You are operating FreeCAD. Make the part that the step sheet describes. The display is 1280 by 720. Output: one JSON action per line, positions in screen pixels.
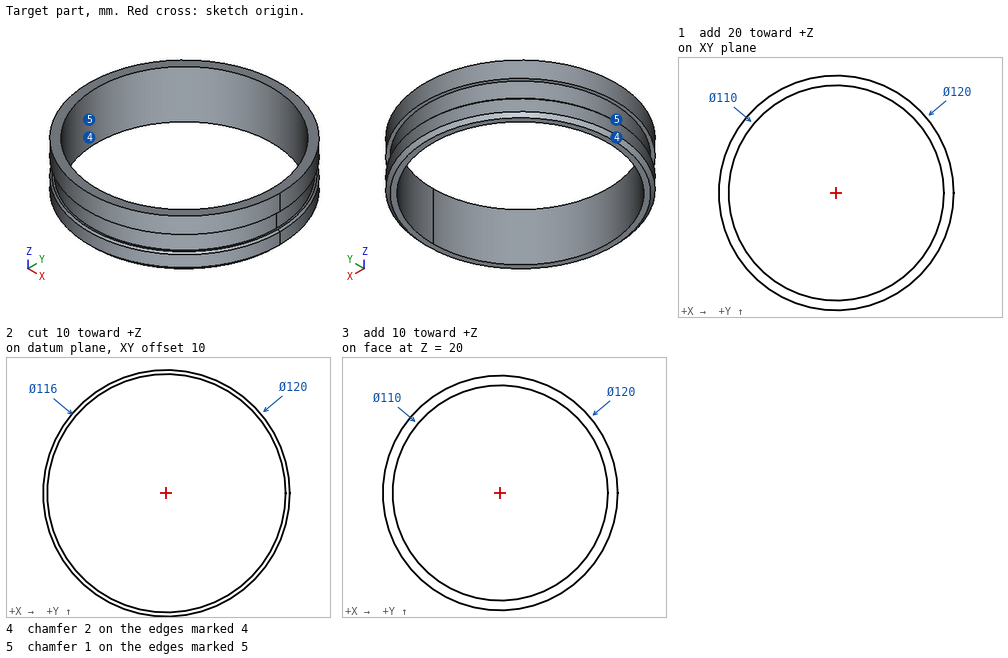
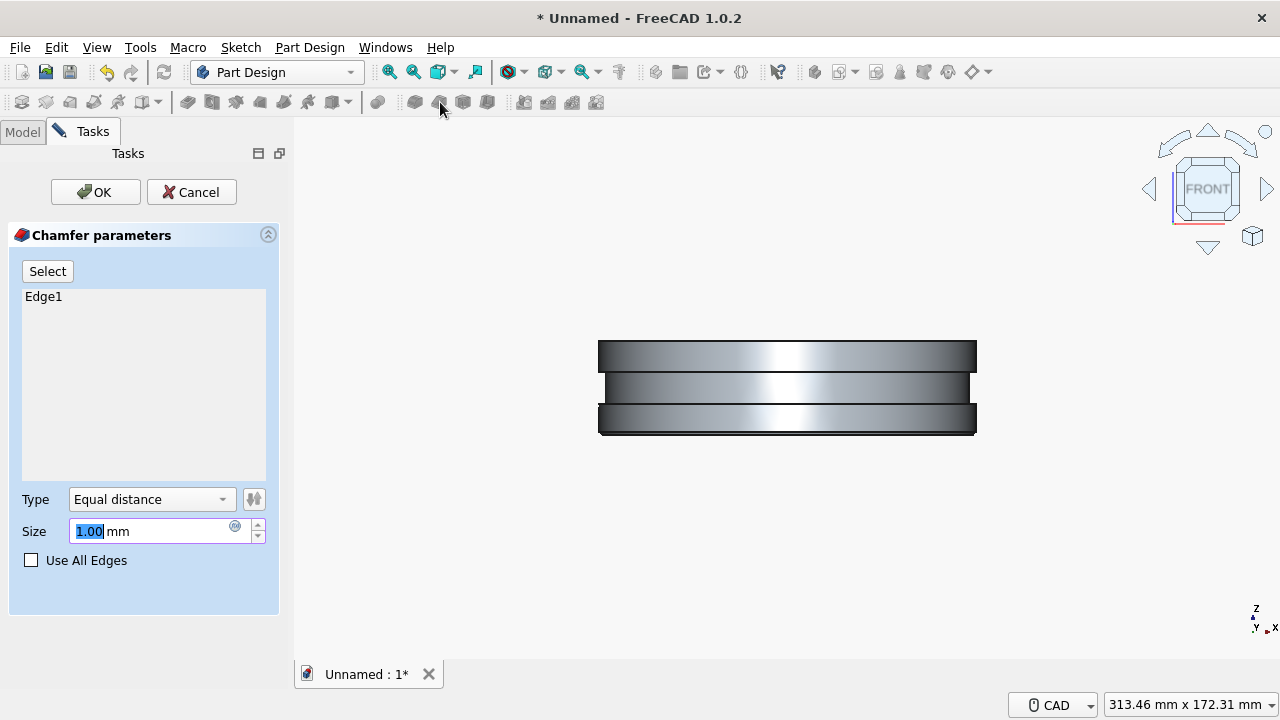
{"action": "type", "text": "2"}
{"action": "key", "text": "Tab"}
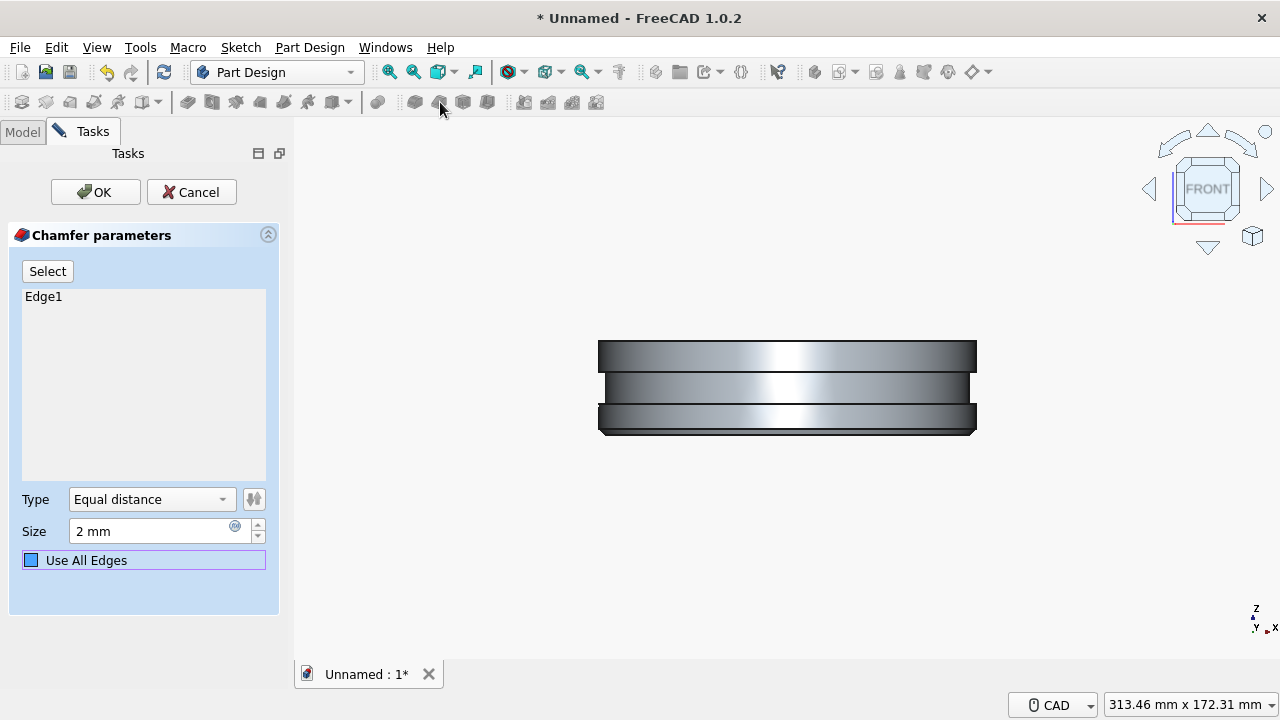
{"action": "left_click", "coordinate": [96, 192]}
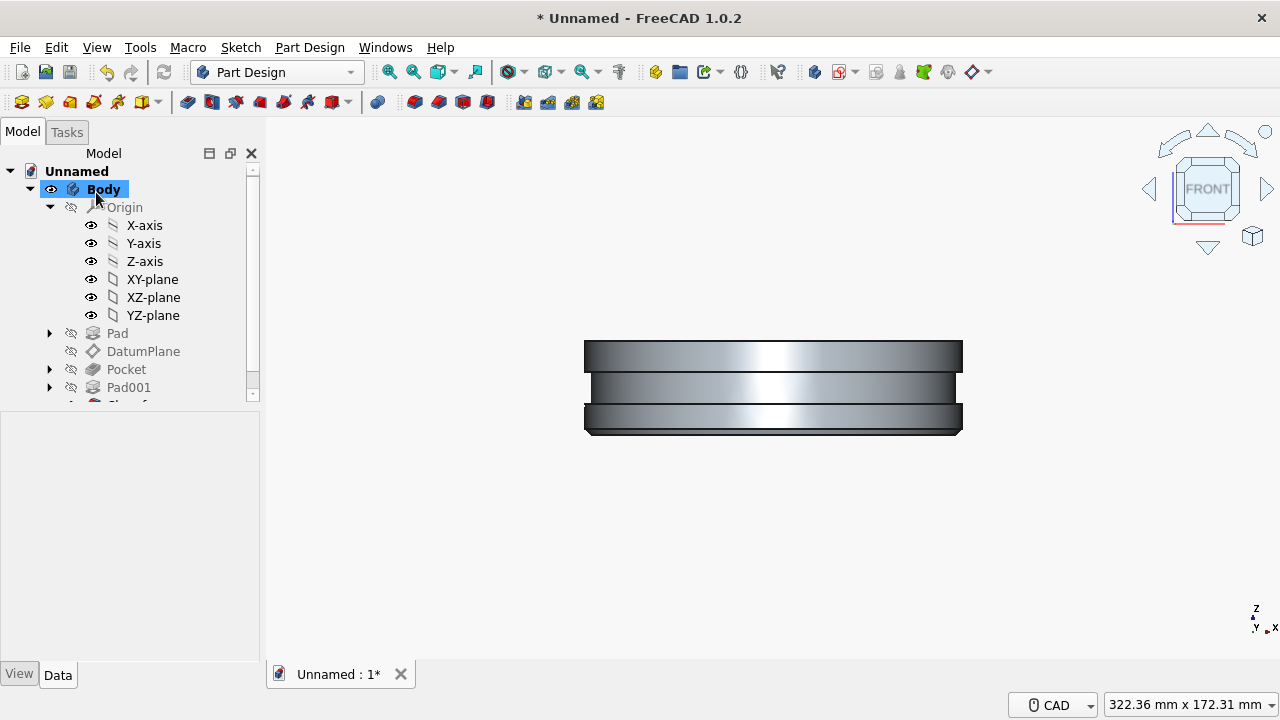
{"action": "key", "text": "v f"}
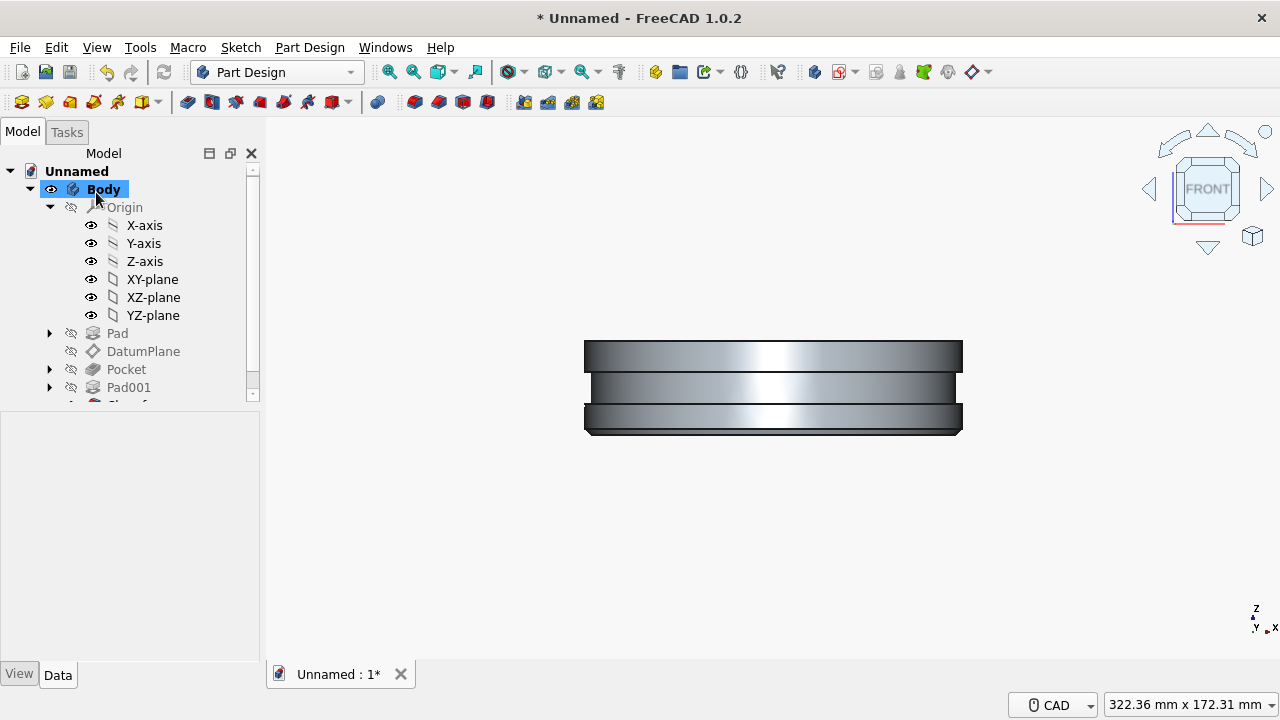
{"action": "left_click", "coordinate": [831, 403]}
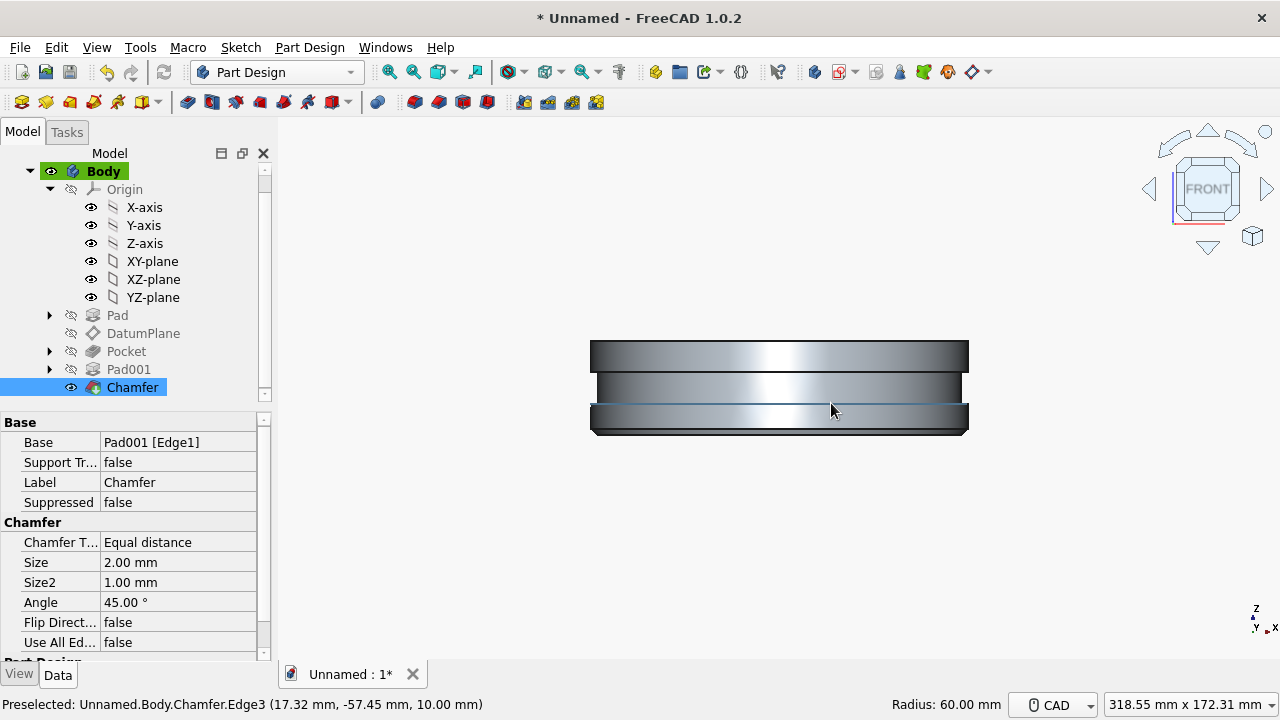
{"action": "left_click", "coordinate": [440, 102]}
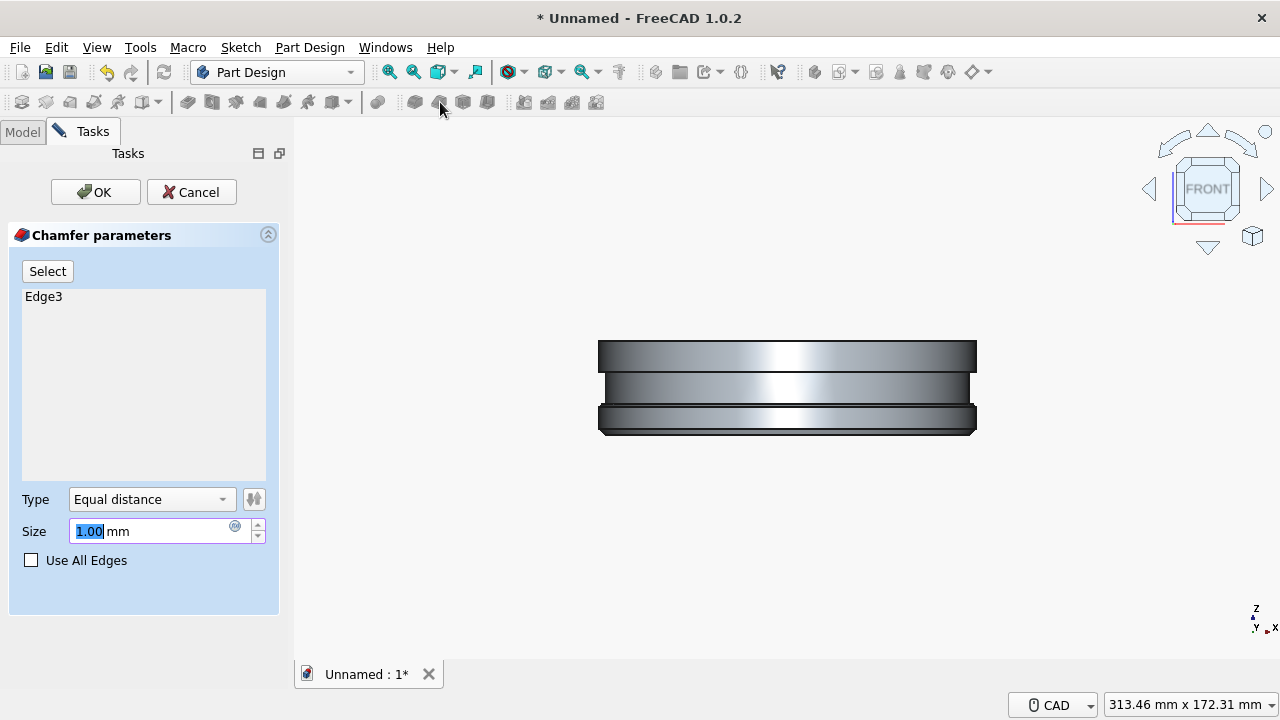
{"action": "type", "text": "1"}
{"action": "key", "text": "Tab"}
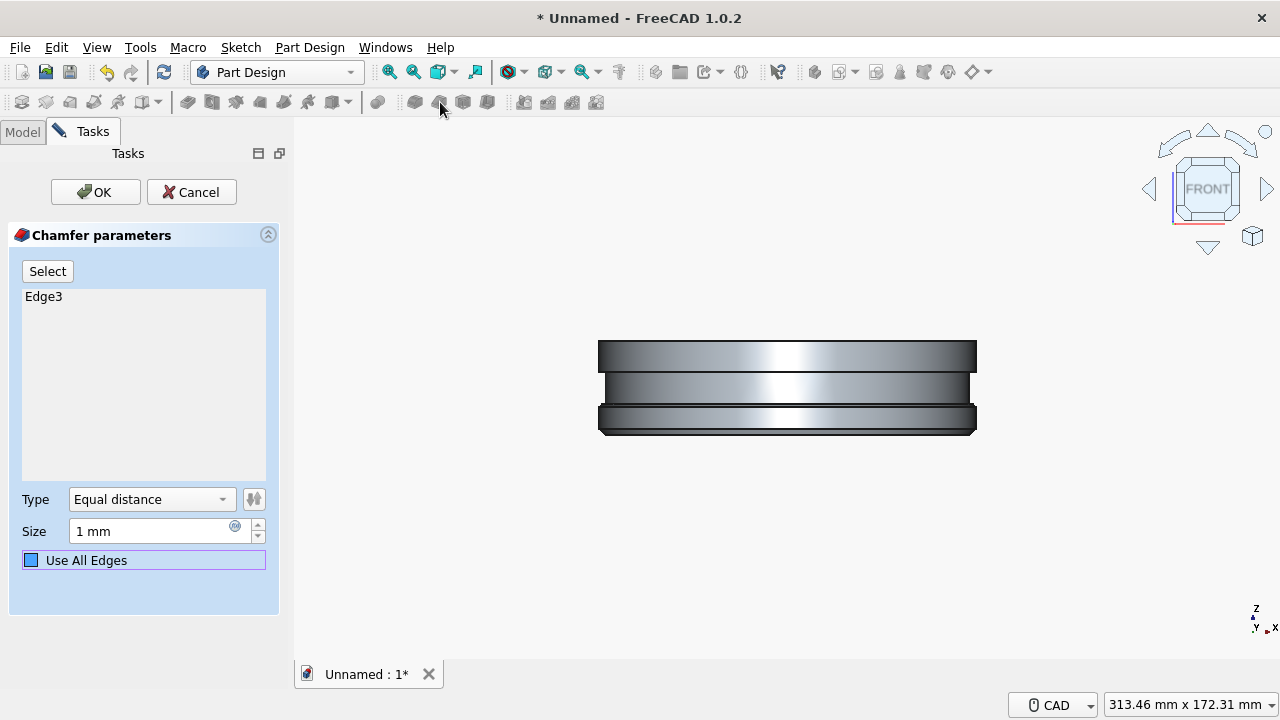
{"action": "left_click", "coordinate": [96, 192]}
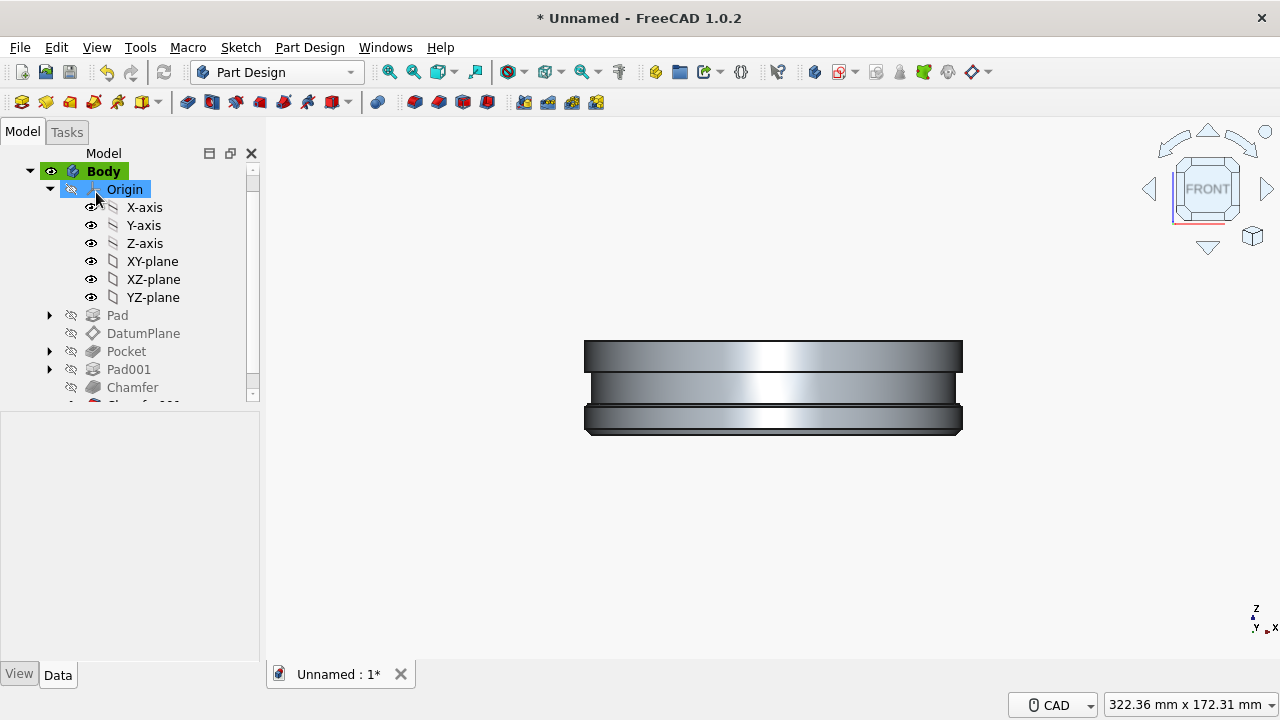
{"action": "key", "text": "0"}